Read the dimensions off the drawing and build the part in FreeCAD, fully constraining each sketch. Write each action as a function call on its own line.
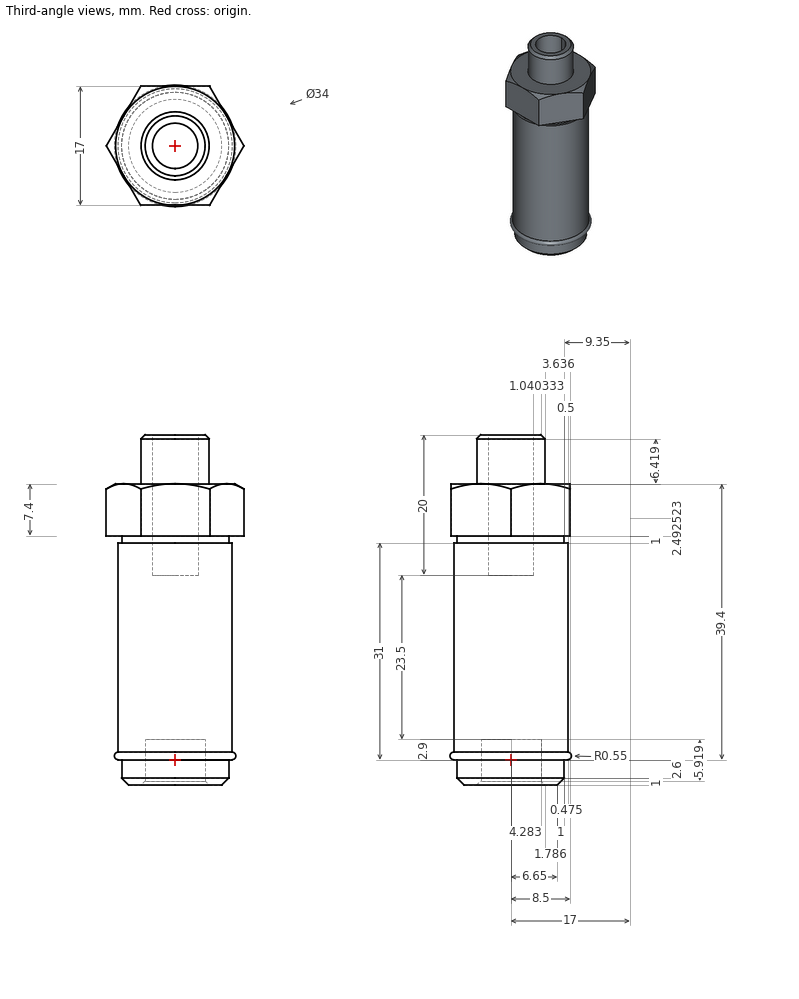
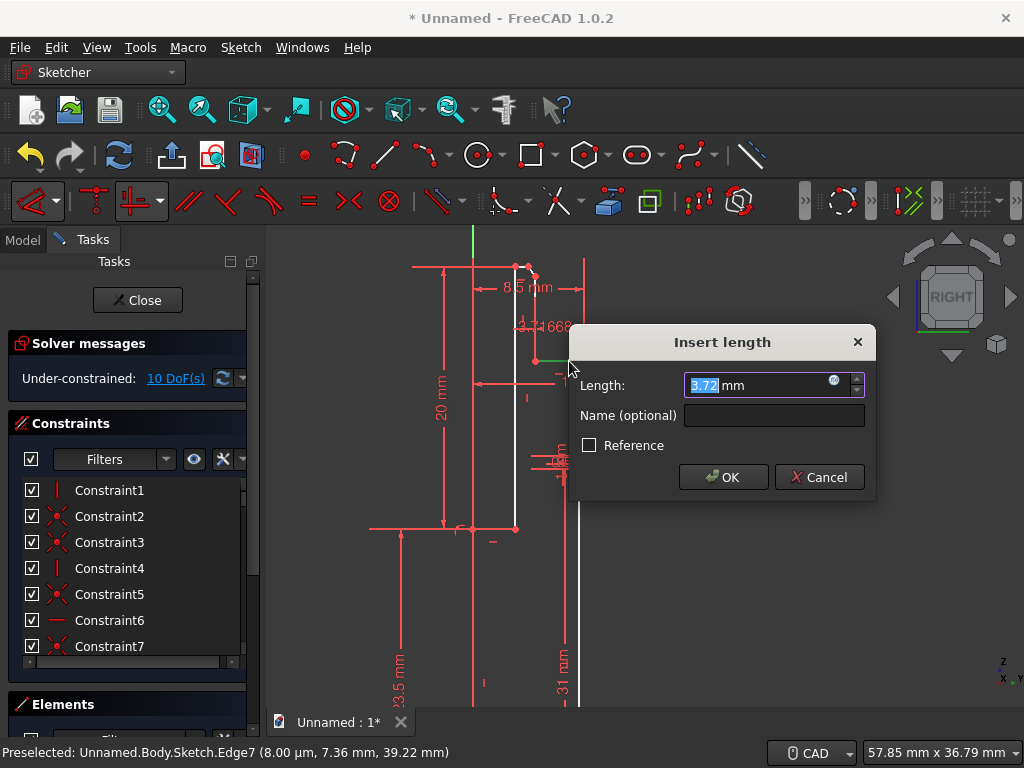
text(3.636)
key(Return)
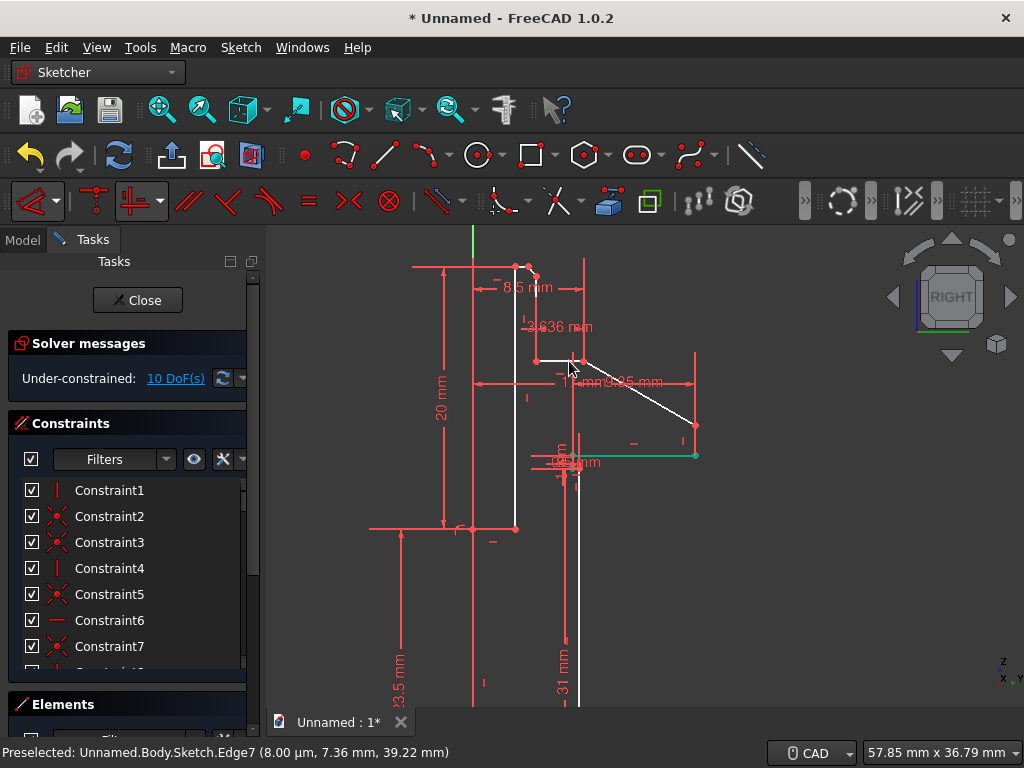
click(536, 336)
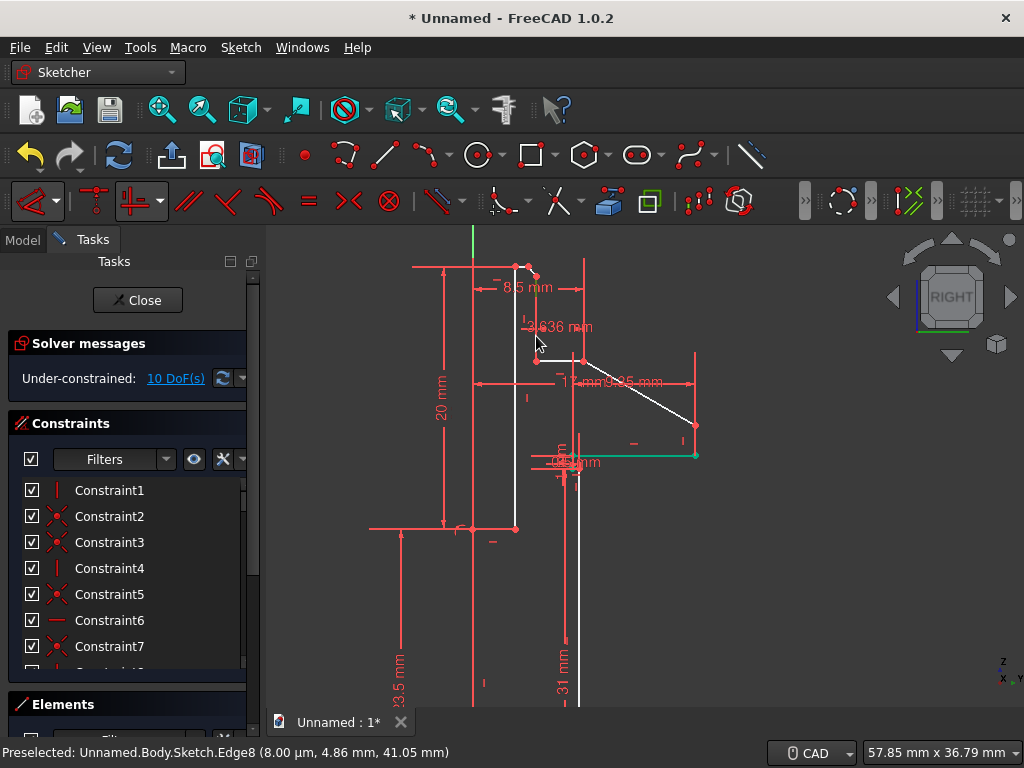
key(i)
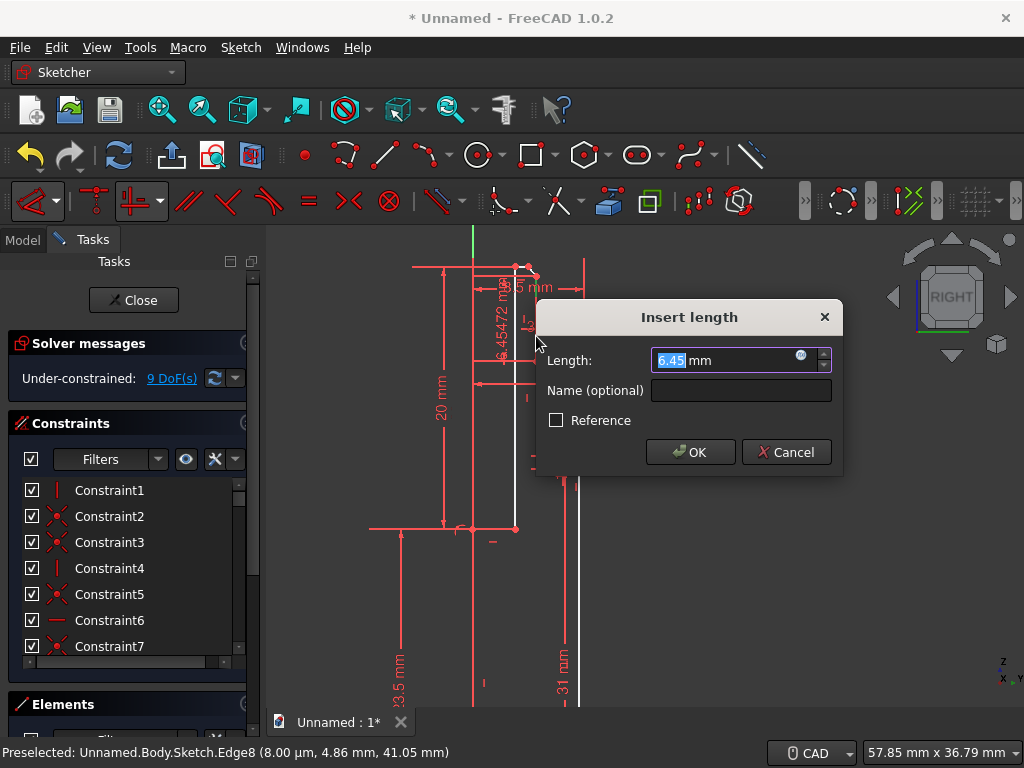
text(6.419)
key(Return)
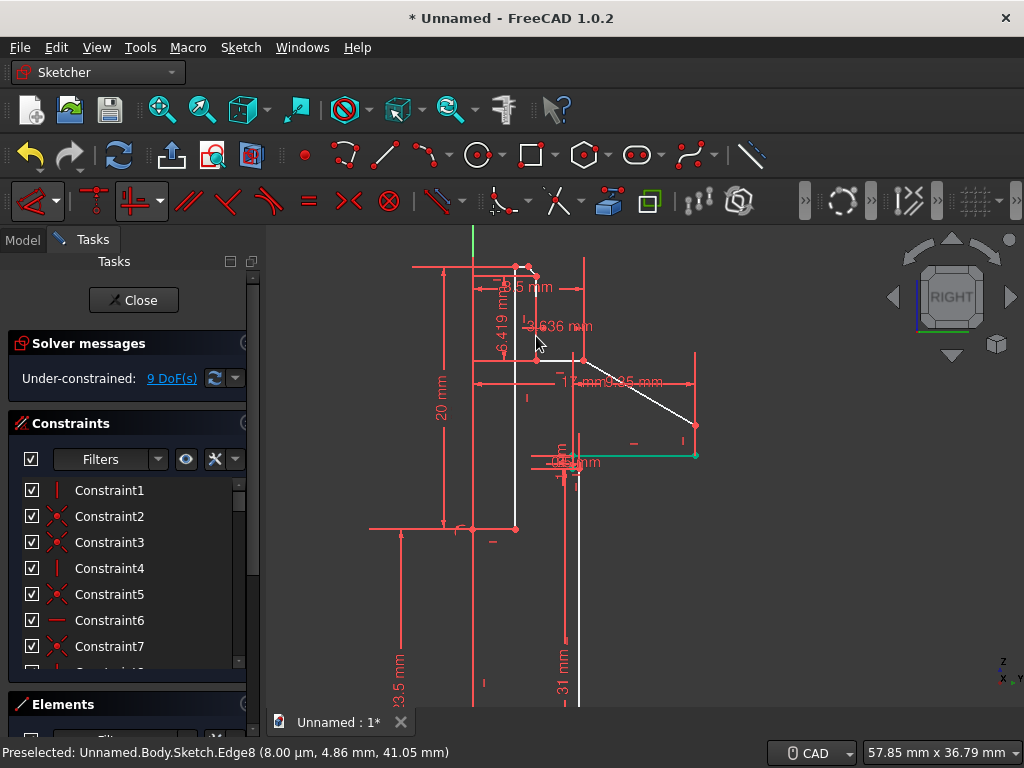
scroll(570, 361, down, 4)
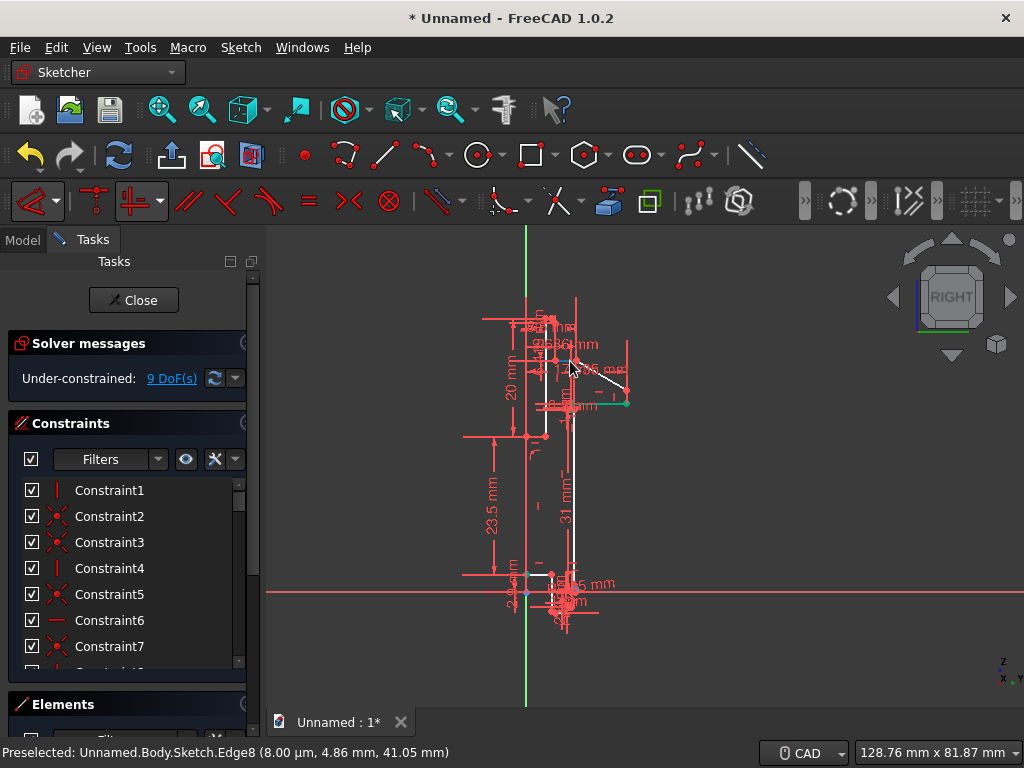
scroll(534, 575, up, 4)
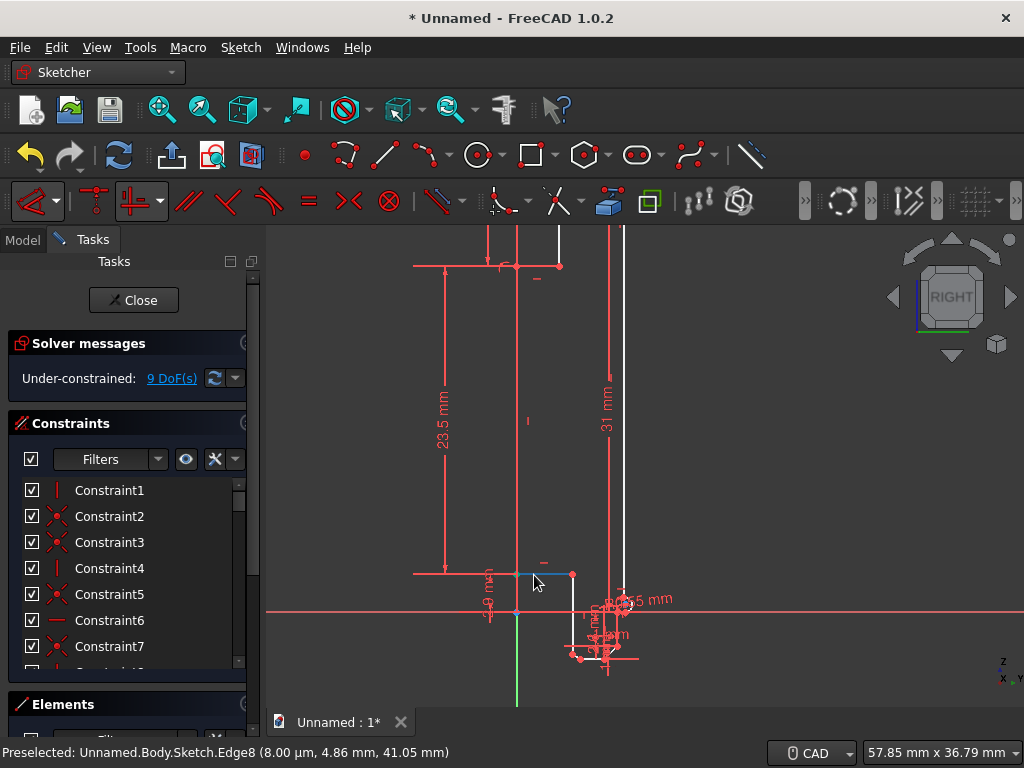
click(534, 574)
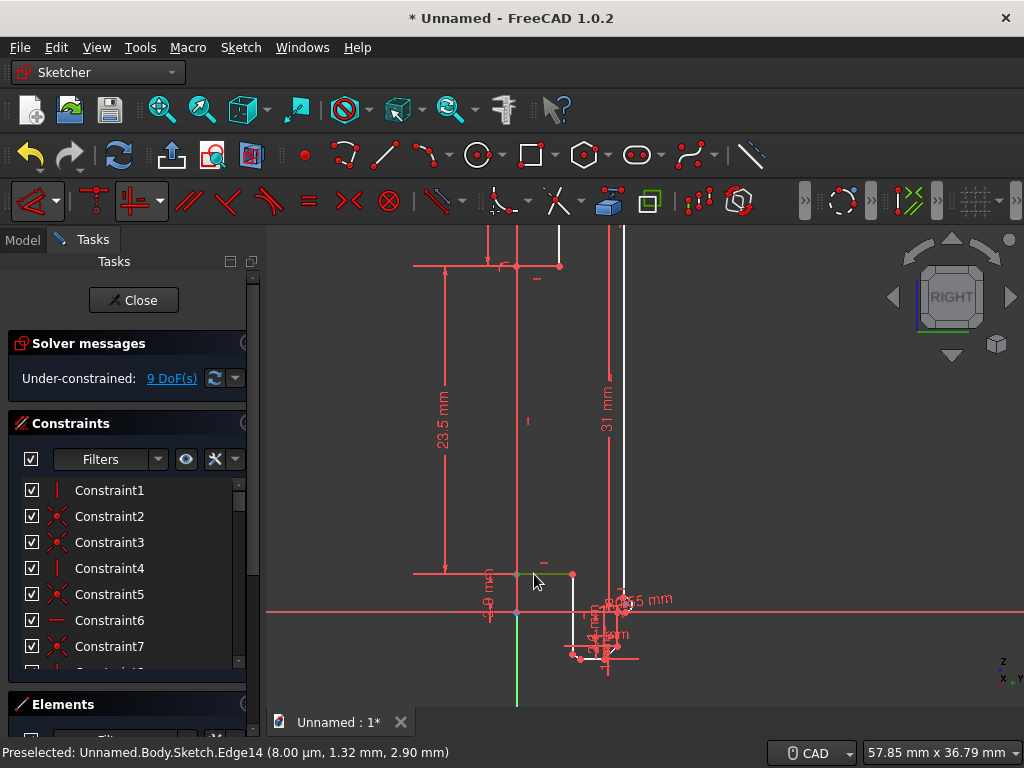
key(l)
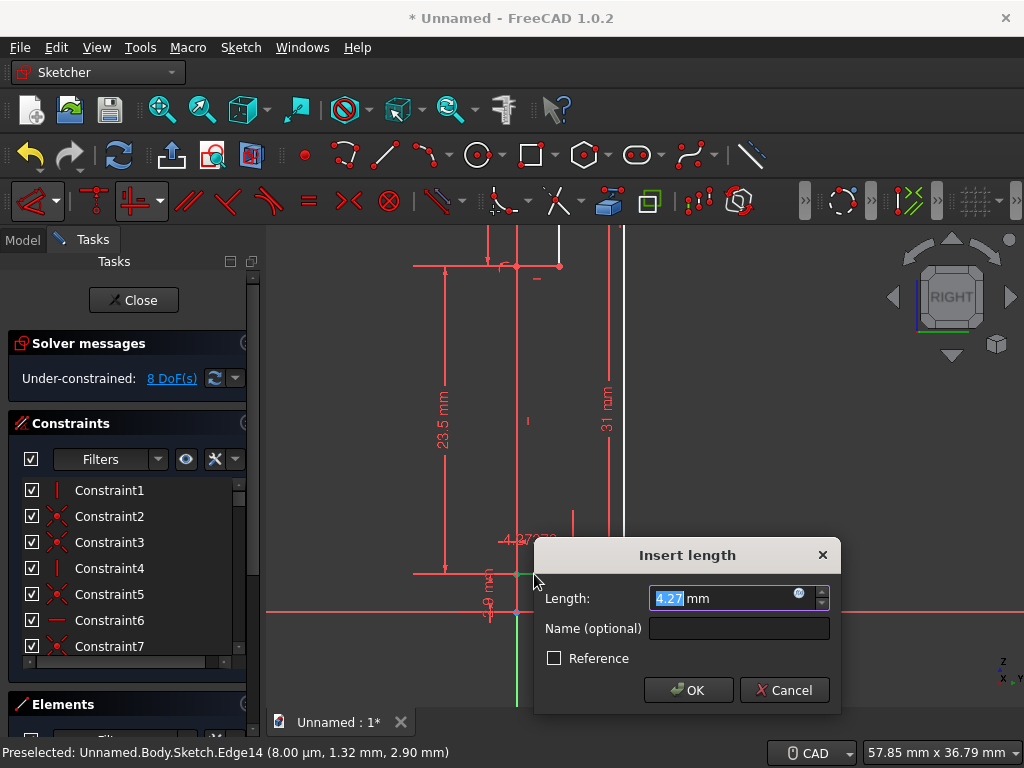
text(4.283)
key(Return)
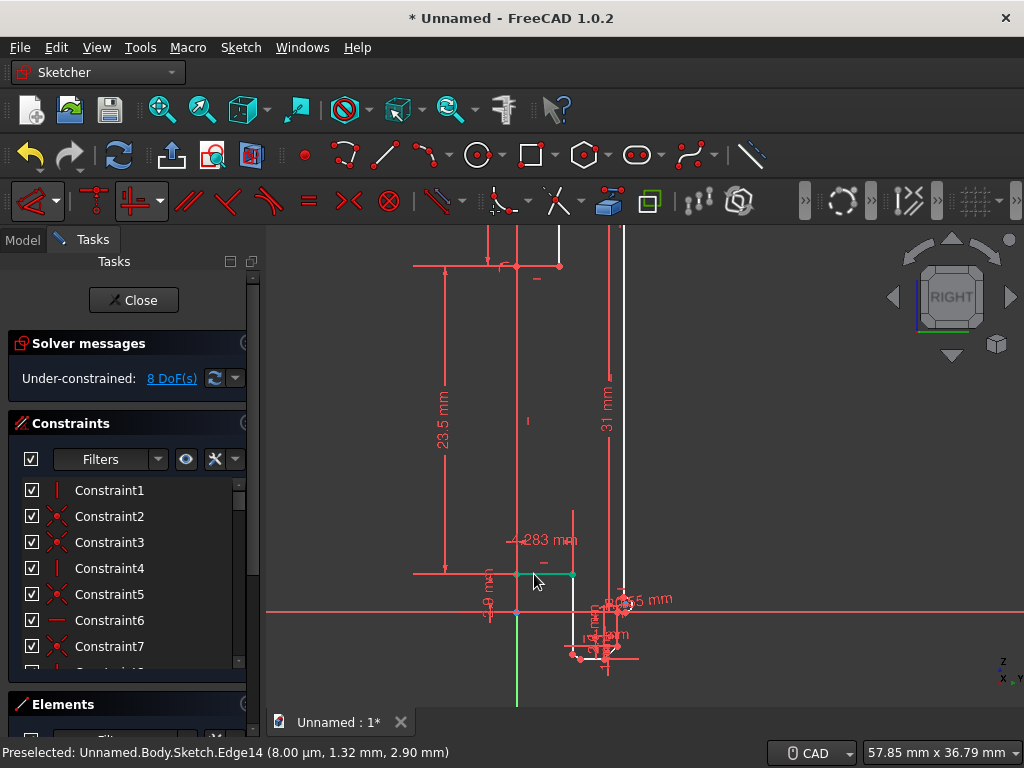
click(573, 598)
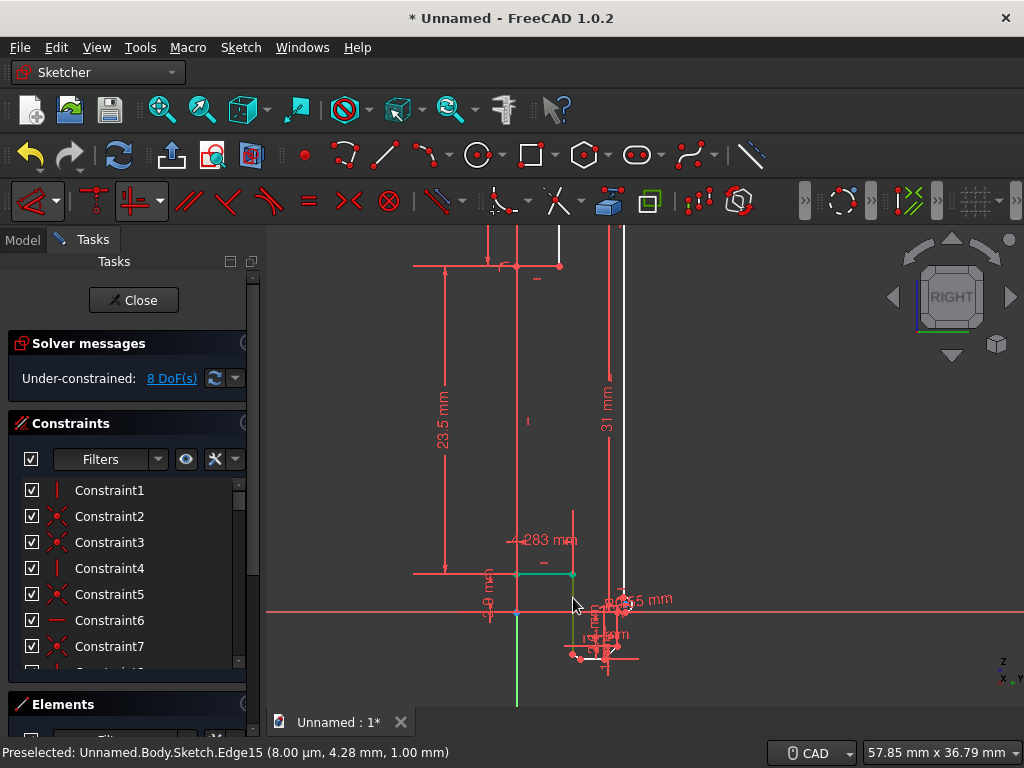
click(58, 202)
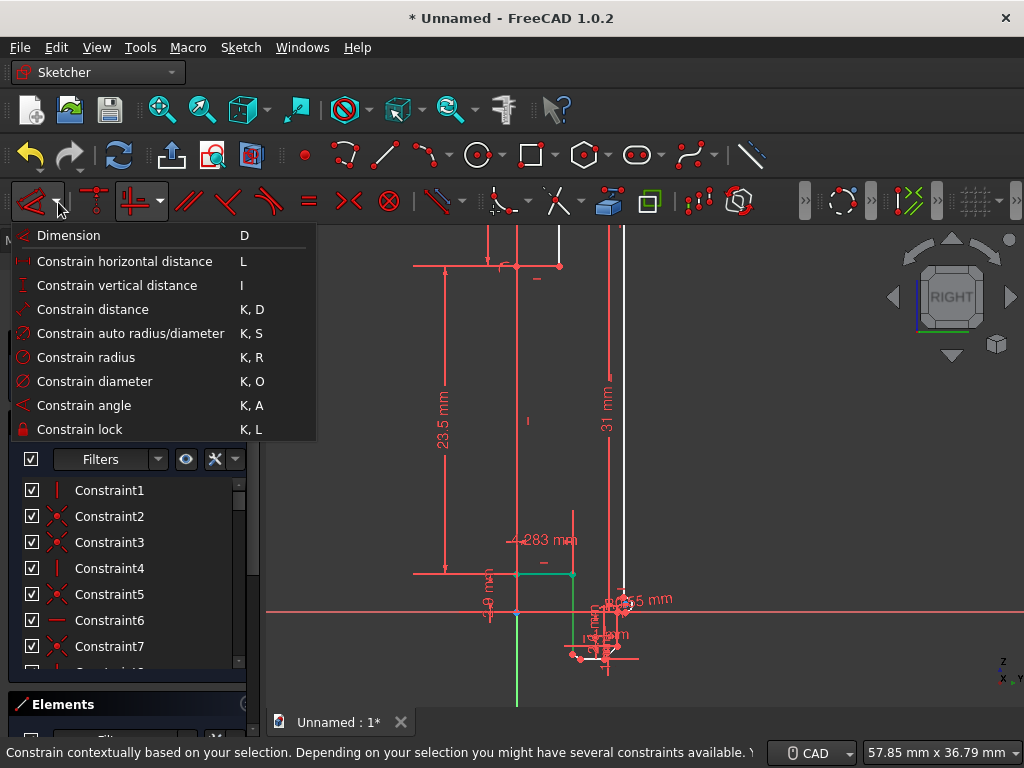
click(164, 285)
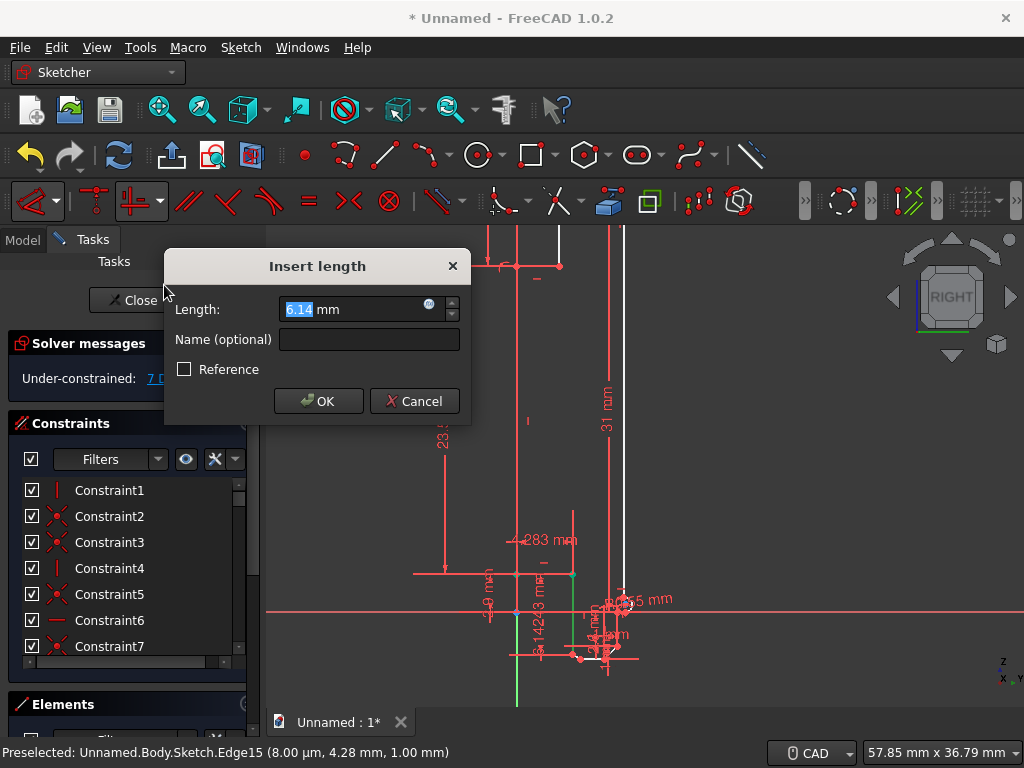
text(5.919)
key(Return)